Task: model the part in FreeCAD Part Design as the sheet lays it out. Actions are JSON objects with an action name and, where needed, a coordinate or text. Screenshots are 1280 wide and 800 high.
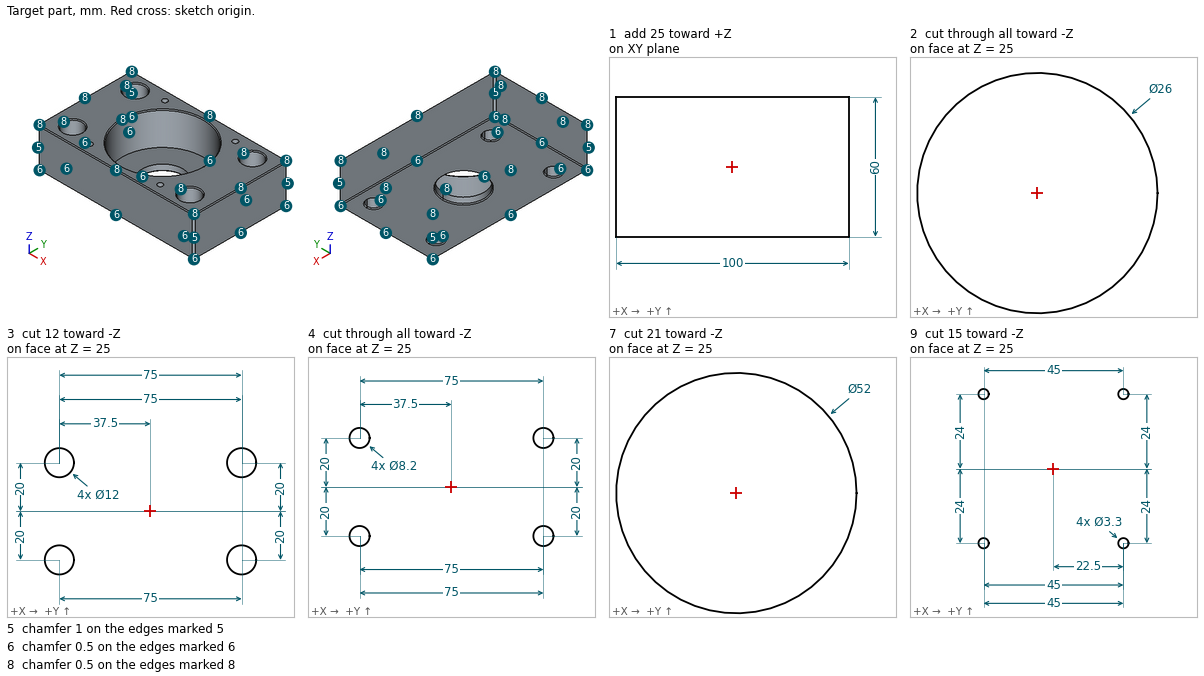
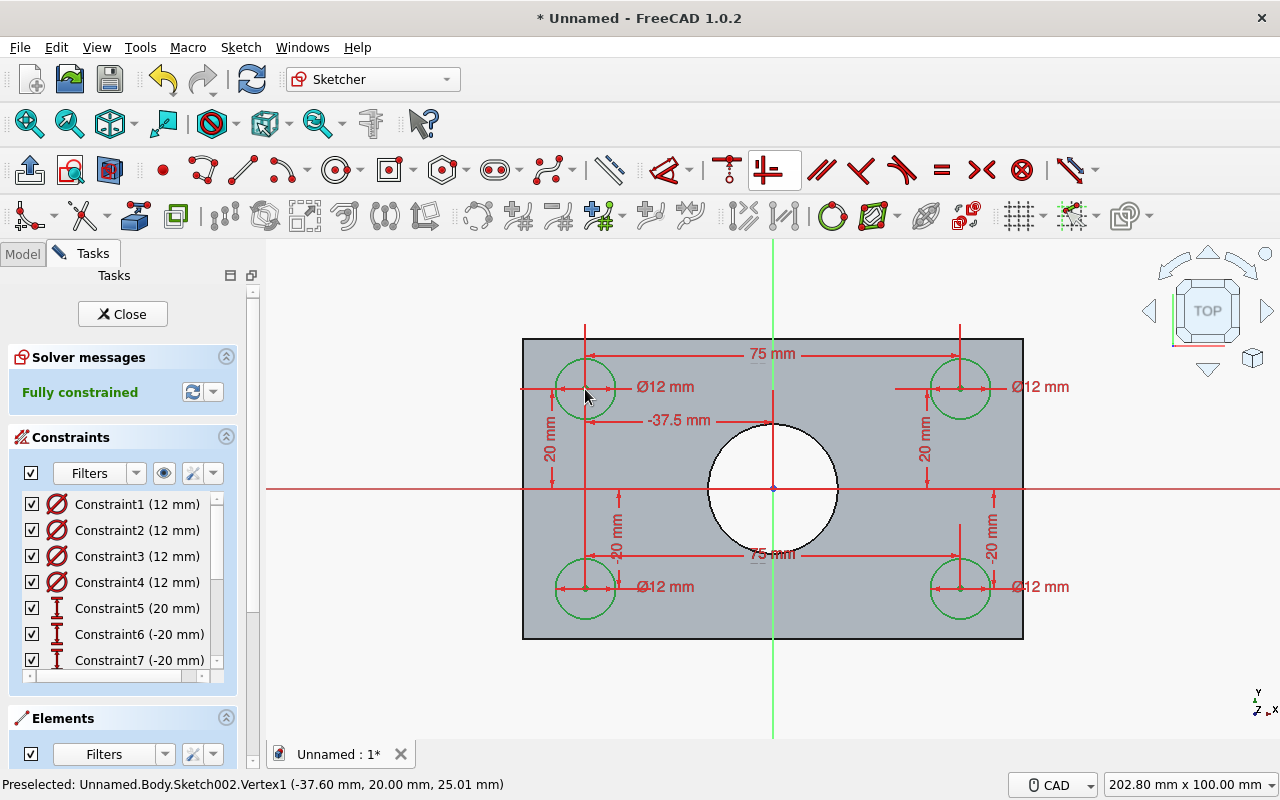
{"action": "left_click", "coordinate": [123, 314]}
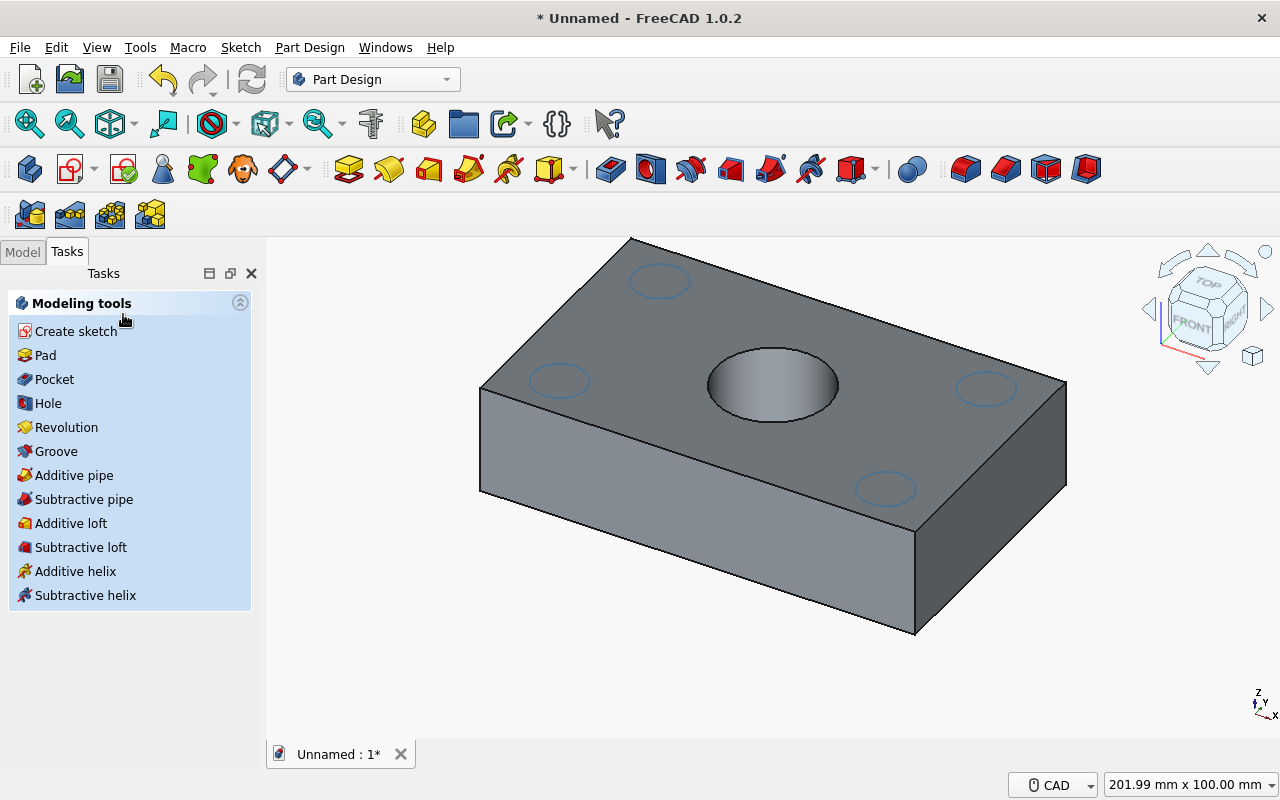
{"action": "left_click", "coordinate": [612, 170]}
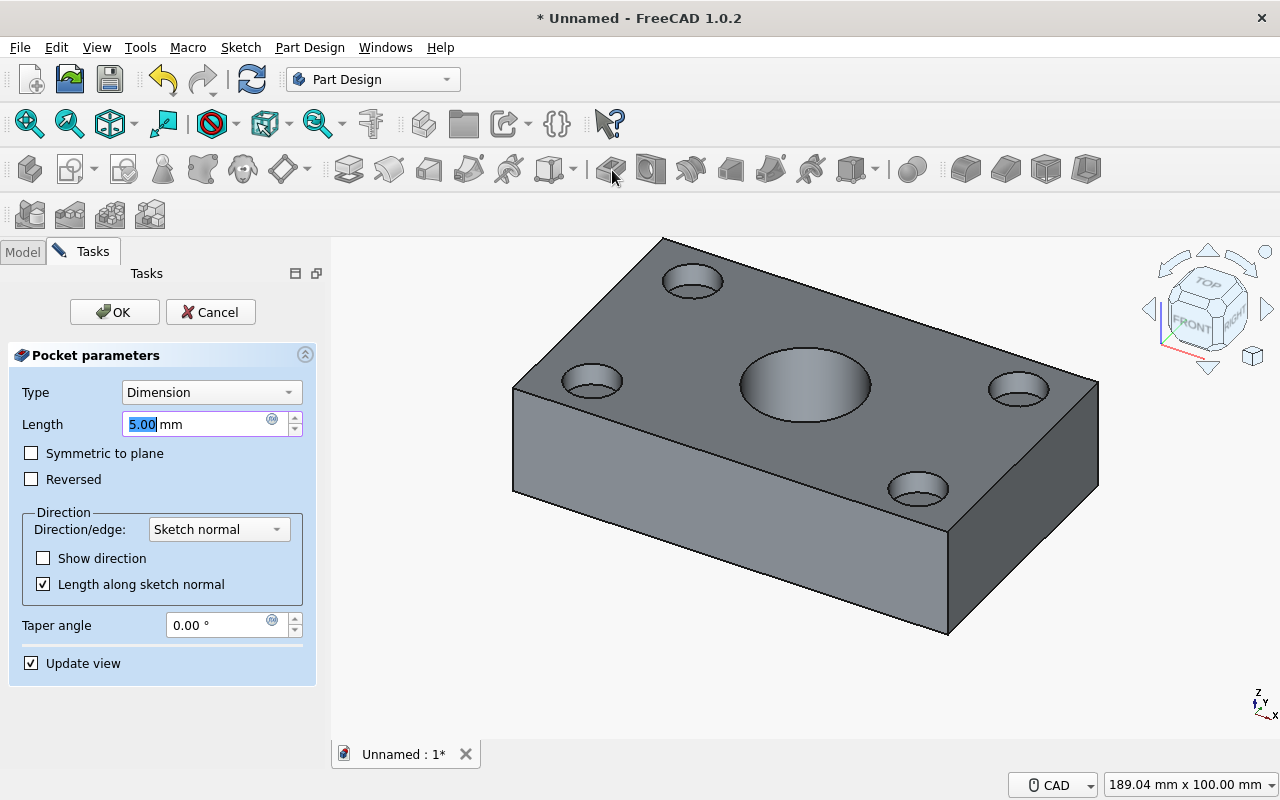
{"action": "type", "text": "12"}
{"action": "key", "text": "Tab"}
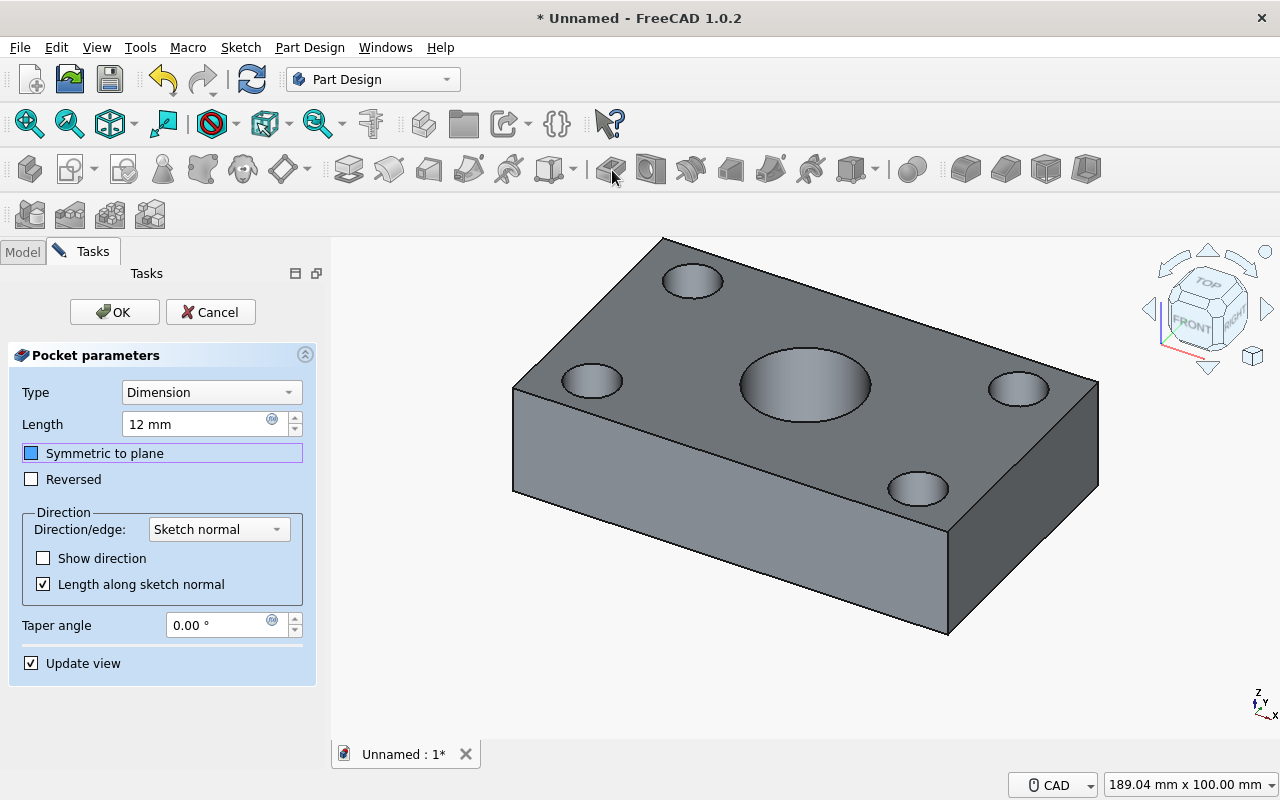
{"action": "left_click", "coordinate": [115, 312]}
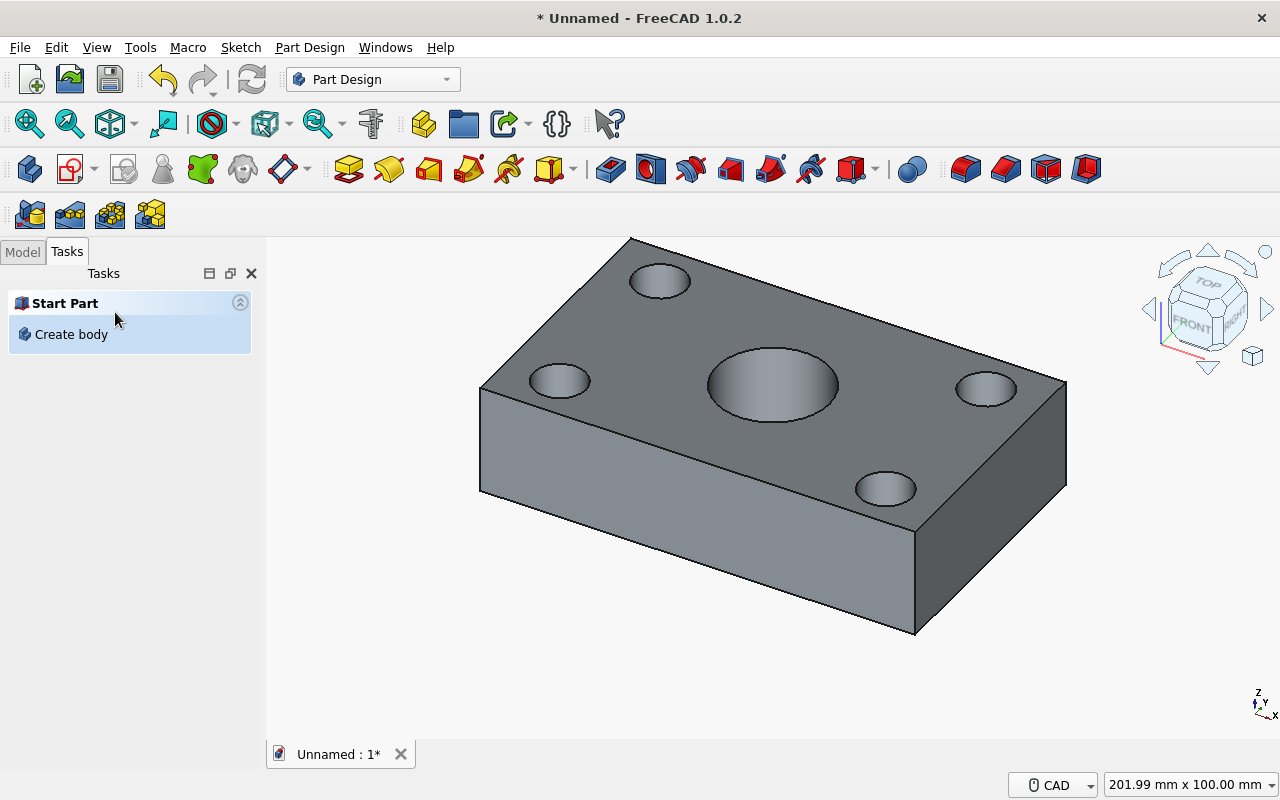
{"action": "left_click", "coordinate": [649, 343]}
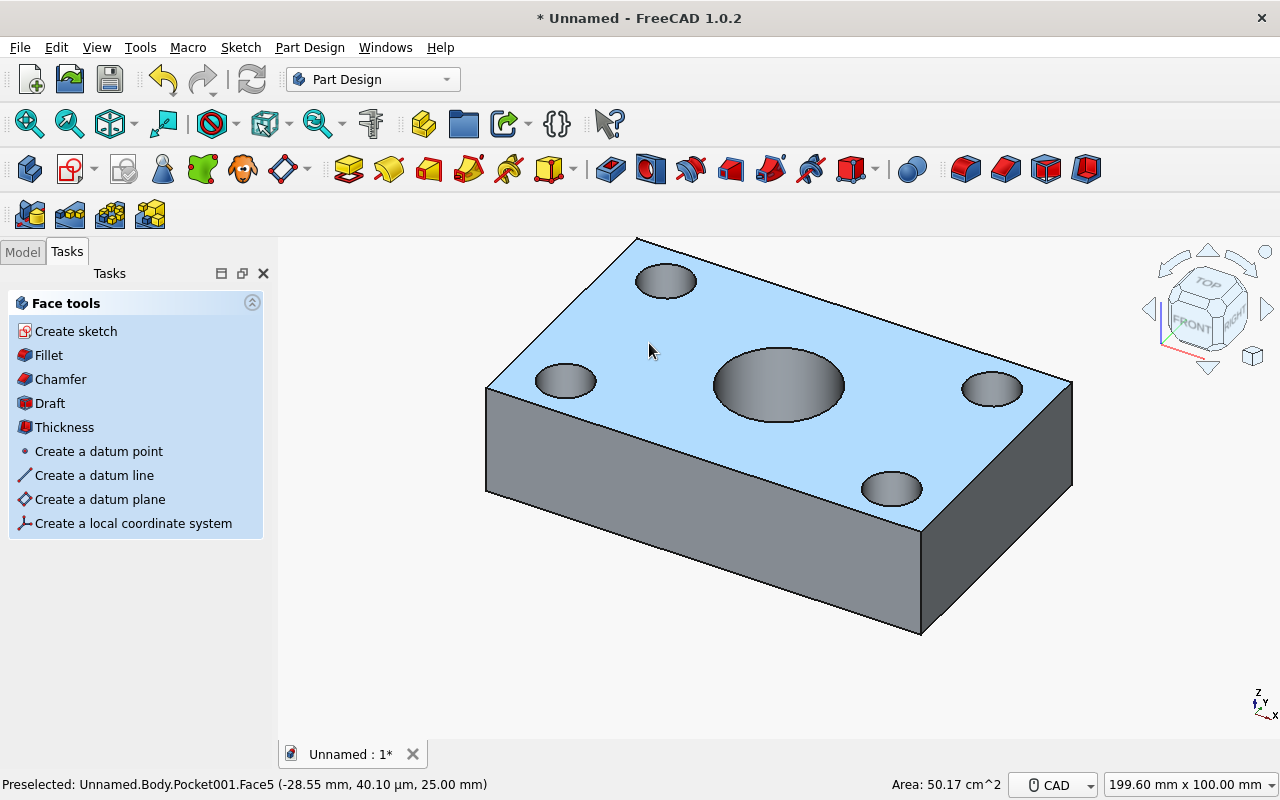
{"action": "left_click", "coordinate": [70, 170]}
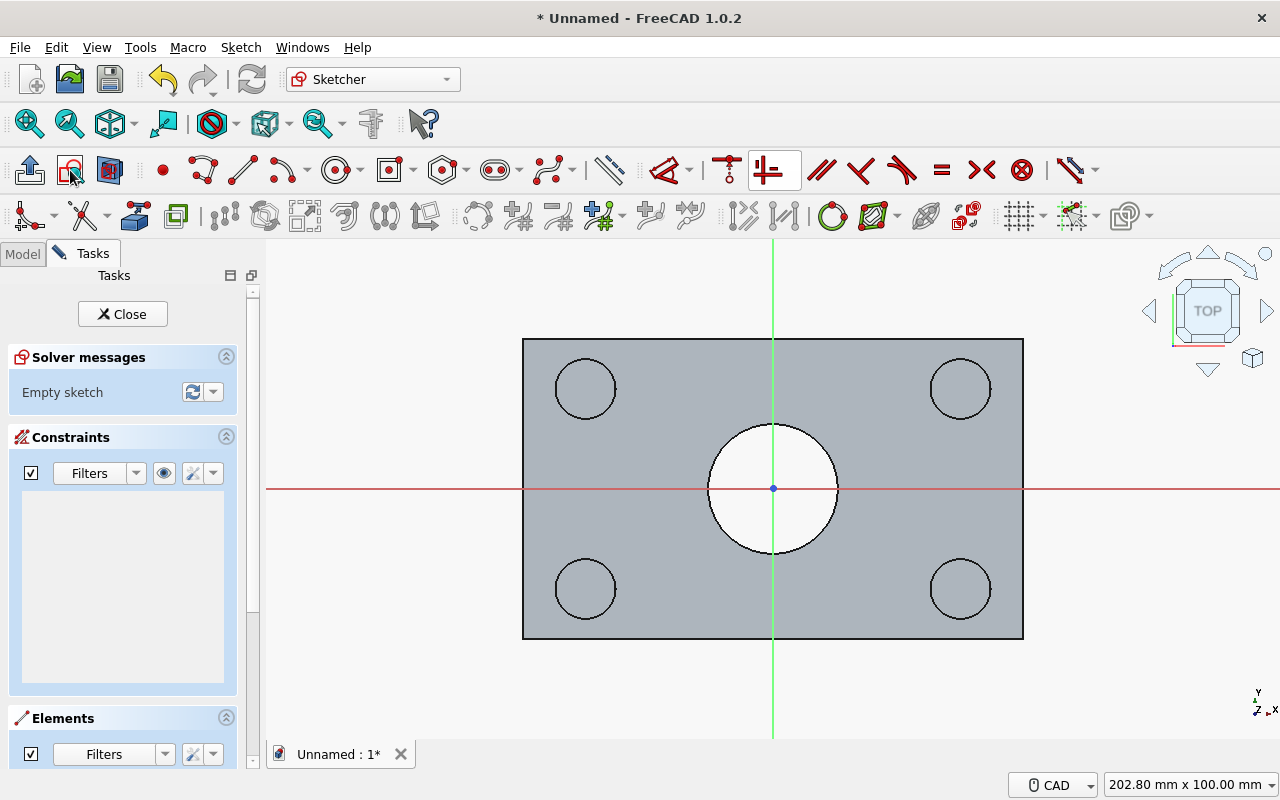
{"action": "key", "text": "g c"}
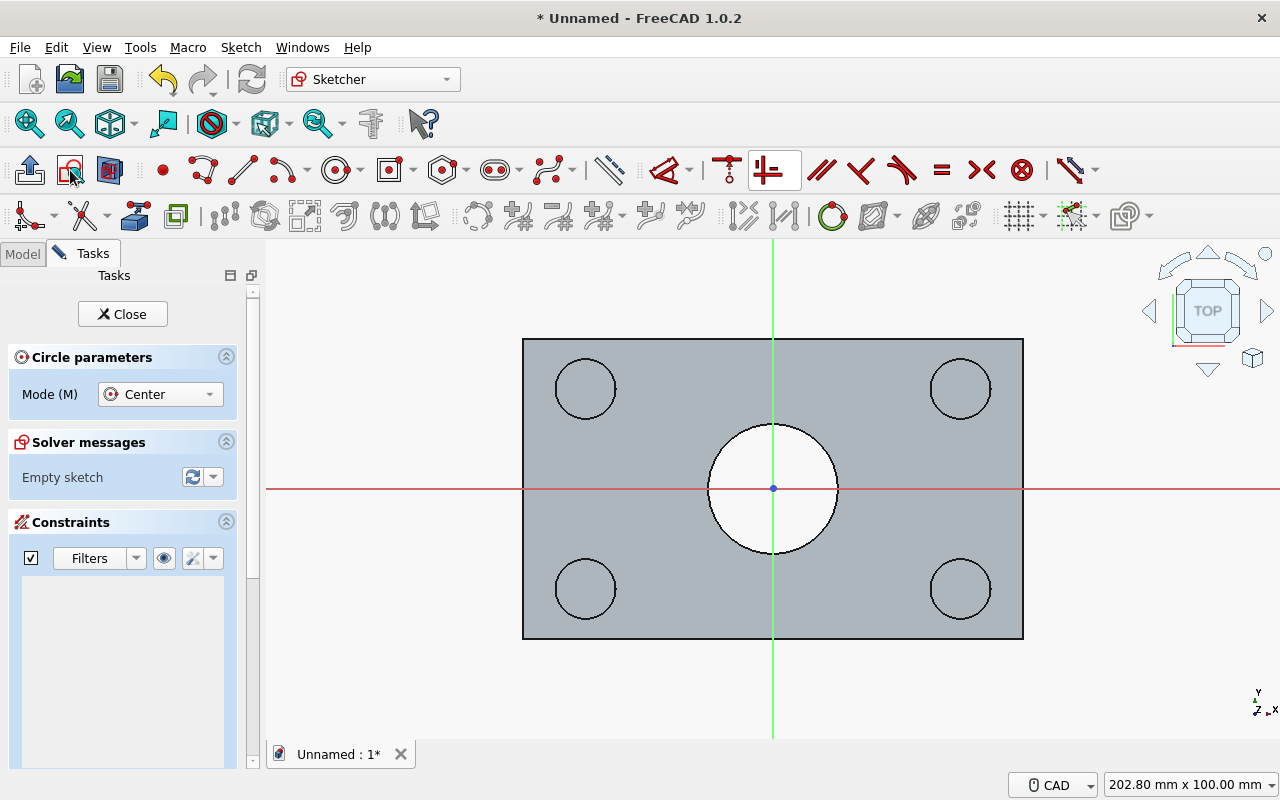
{"action": "left_click", "coordinate": [585, 389]}
{"action": "mouse_move", "coordinate": [600, 375]}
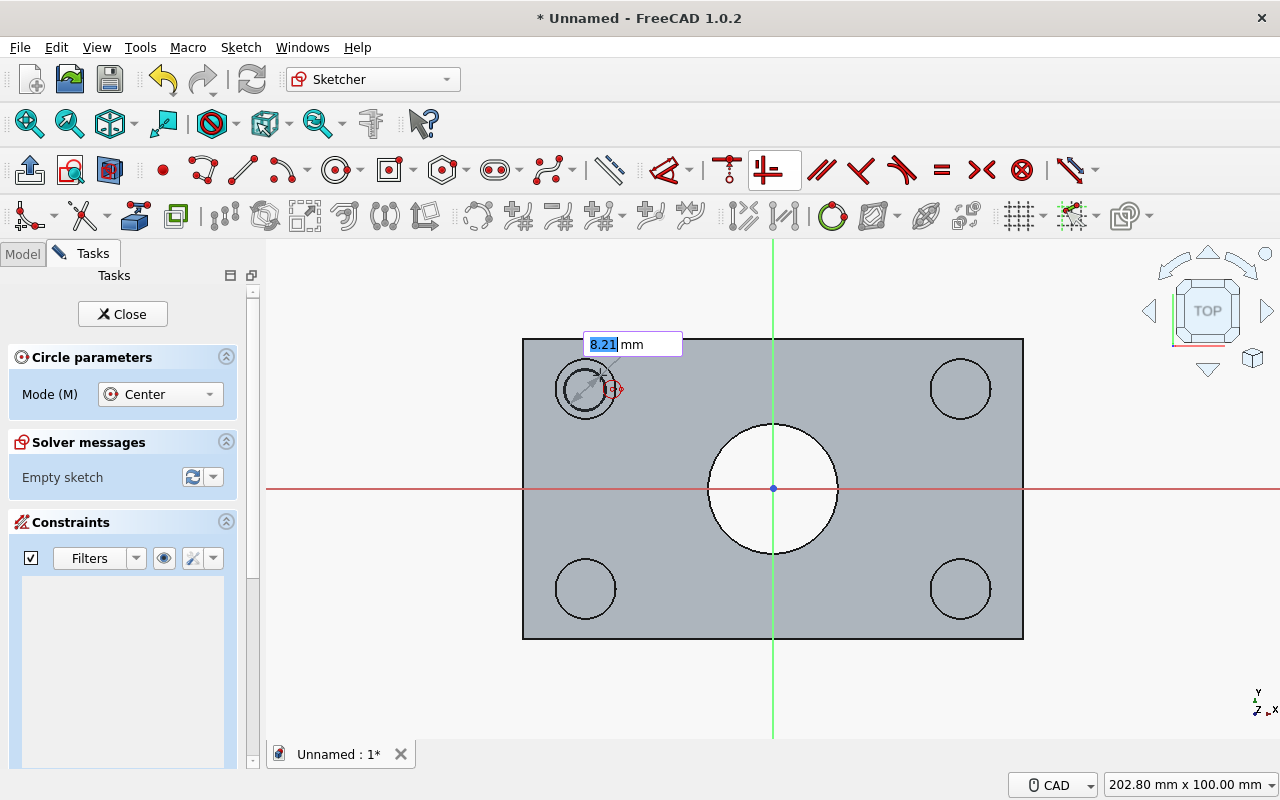
{"action": "type", "text": "8.2"}
{"action": "key", "text": "Return"}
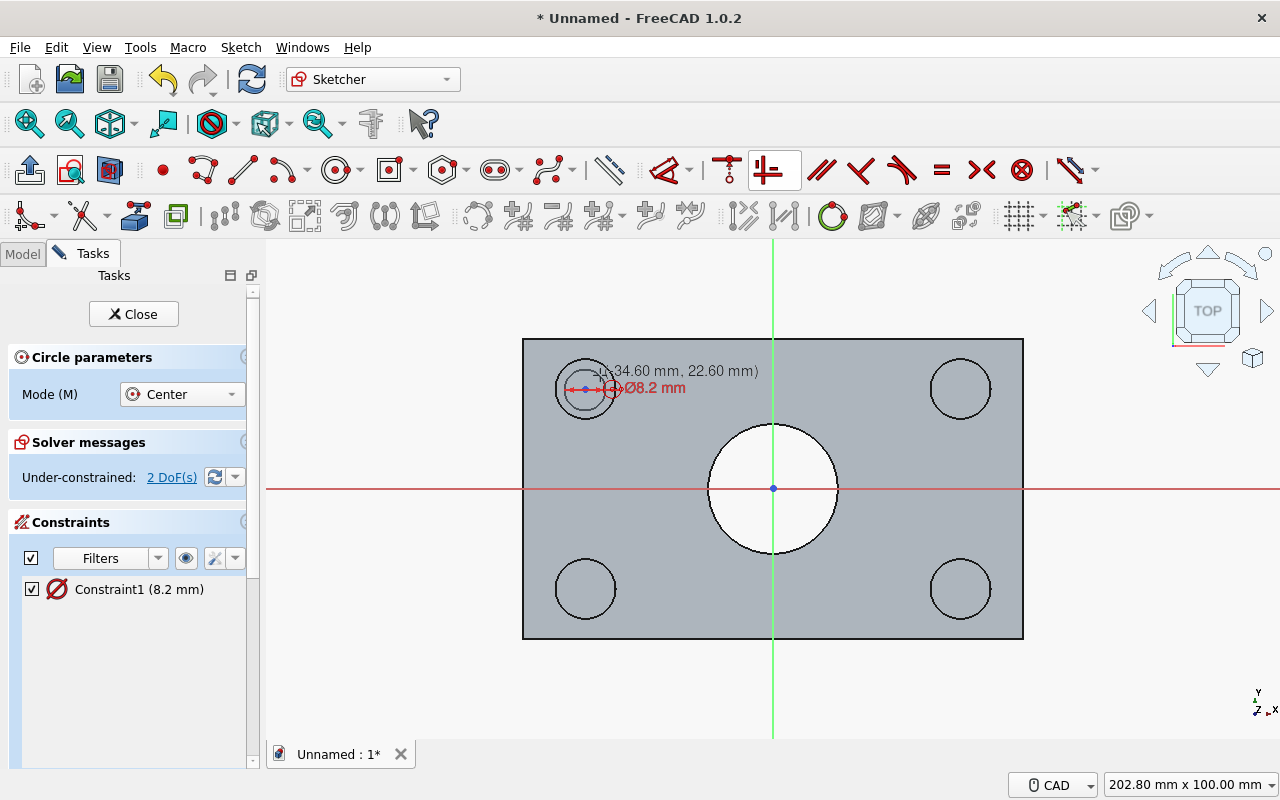
{"action": "left_click", "coordinate": [585, 589]}
{"action": "mouse_move", "coordinate": [600, 575]}